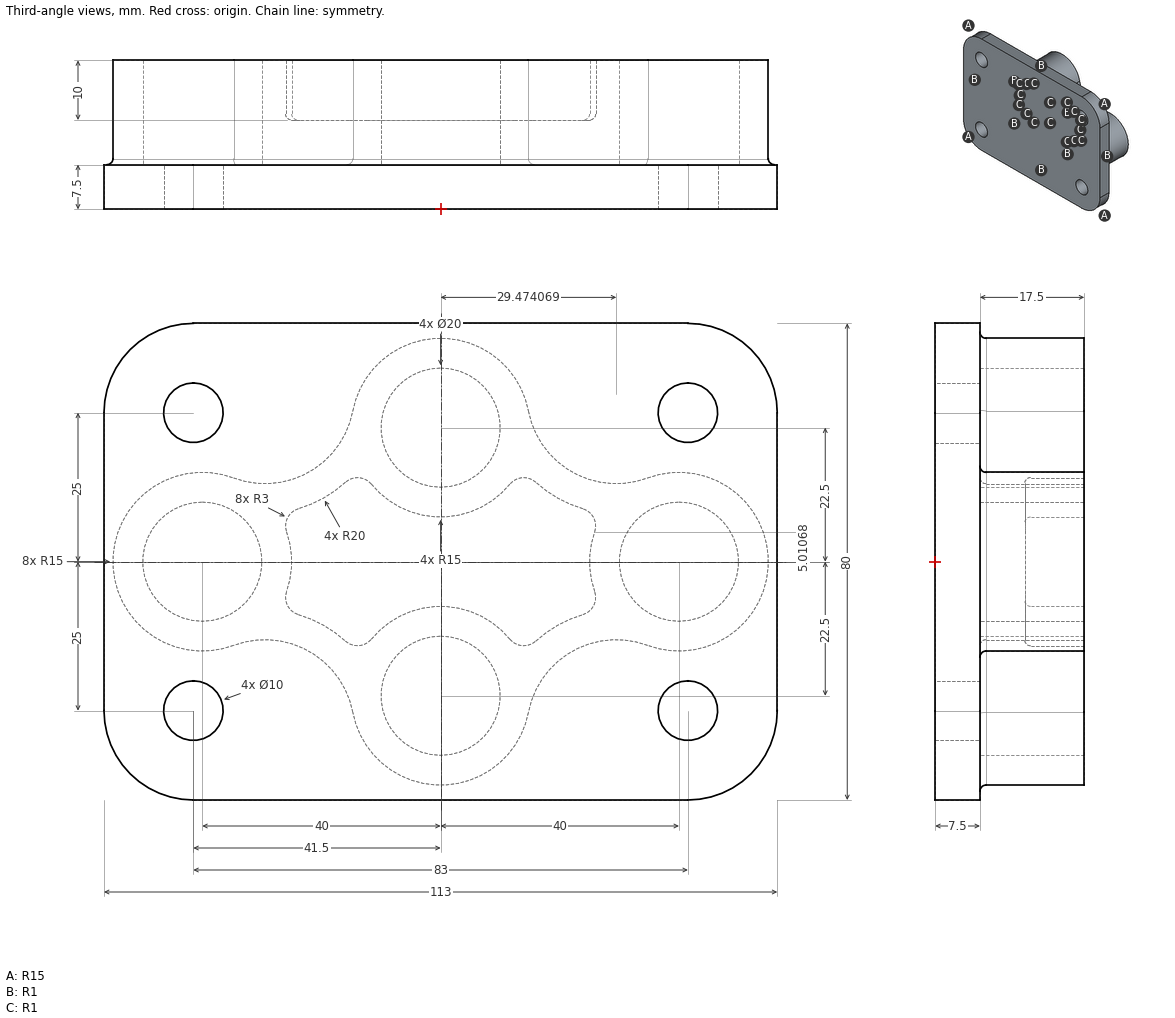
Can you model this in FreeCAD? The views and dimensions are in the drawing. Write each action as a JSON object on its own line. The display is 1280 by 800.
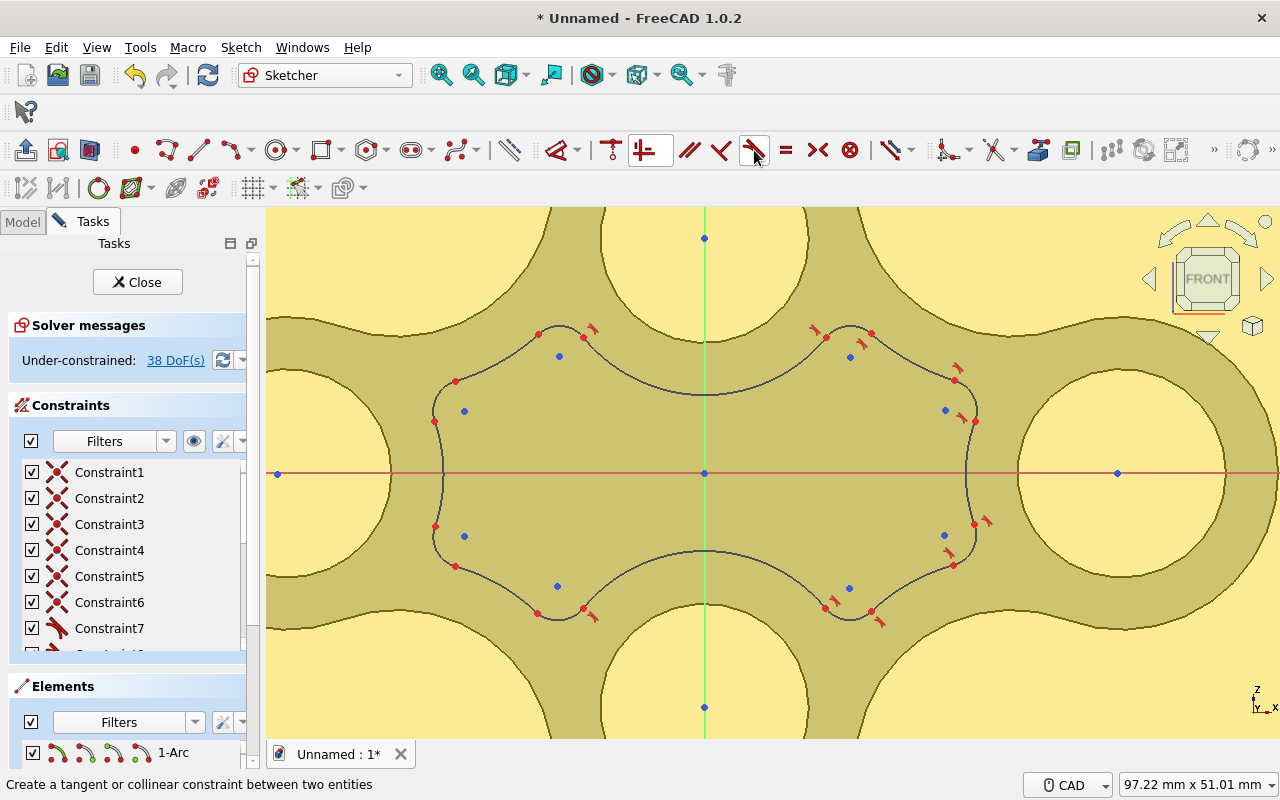
{"action": "left_click", "coordinate": [552, 620]}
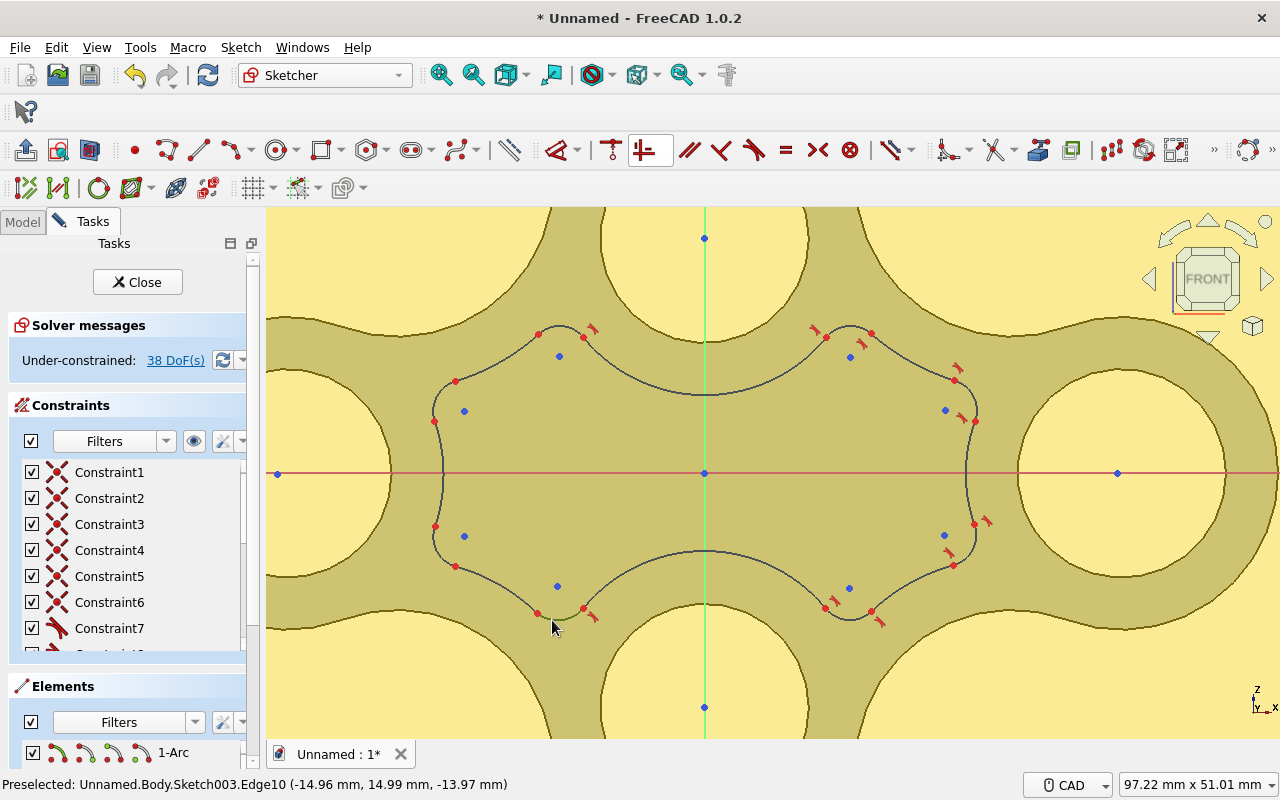
{"action": "left_click", "coordinate": [516, 595]}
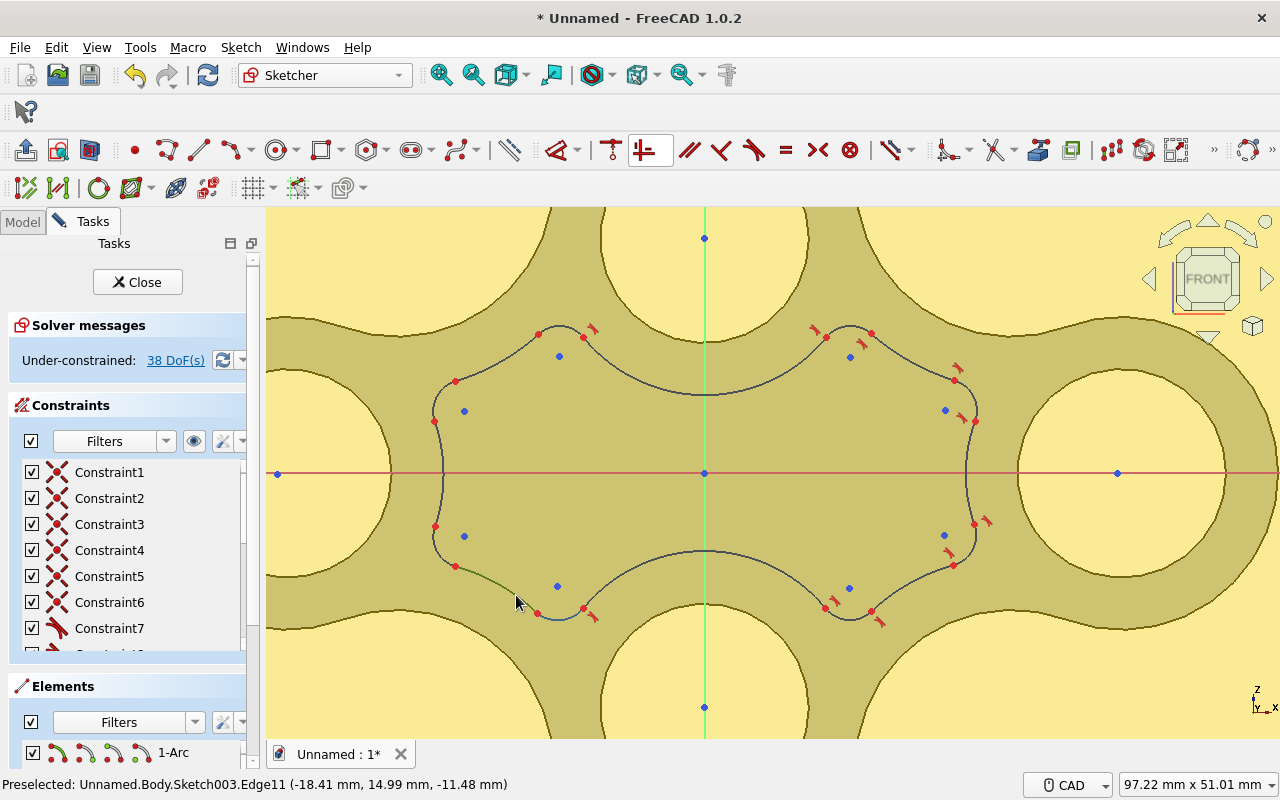
{"action": "key", "text": "t"}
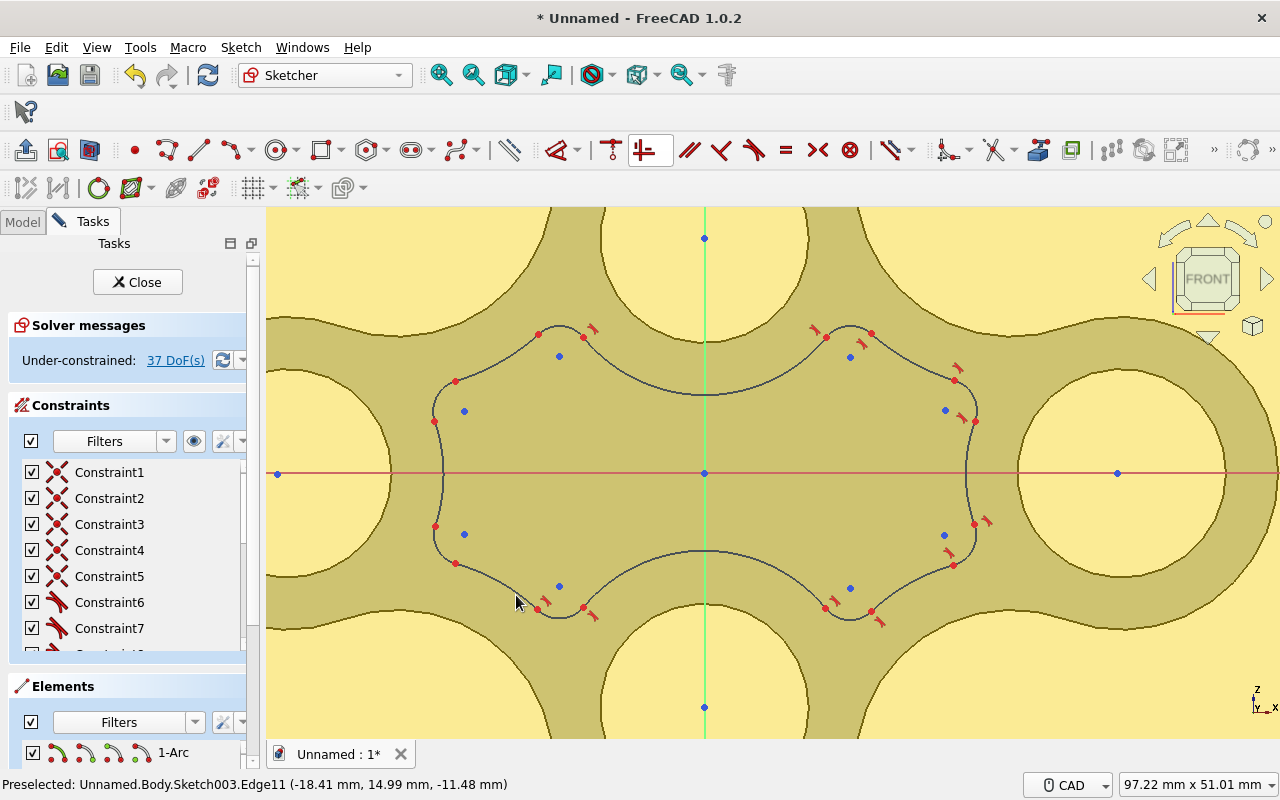
{"action": "left_click", "coordinate": [515, 592]}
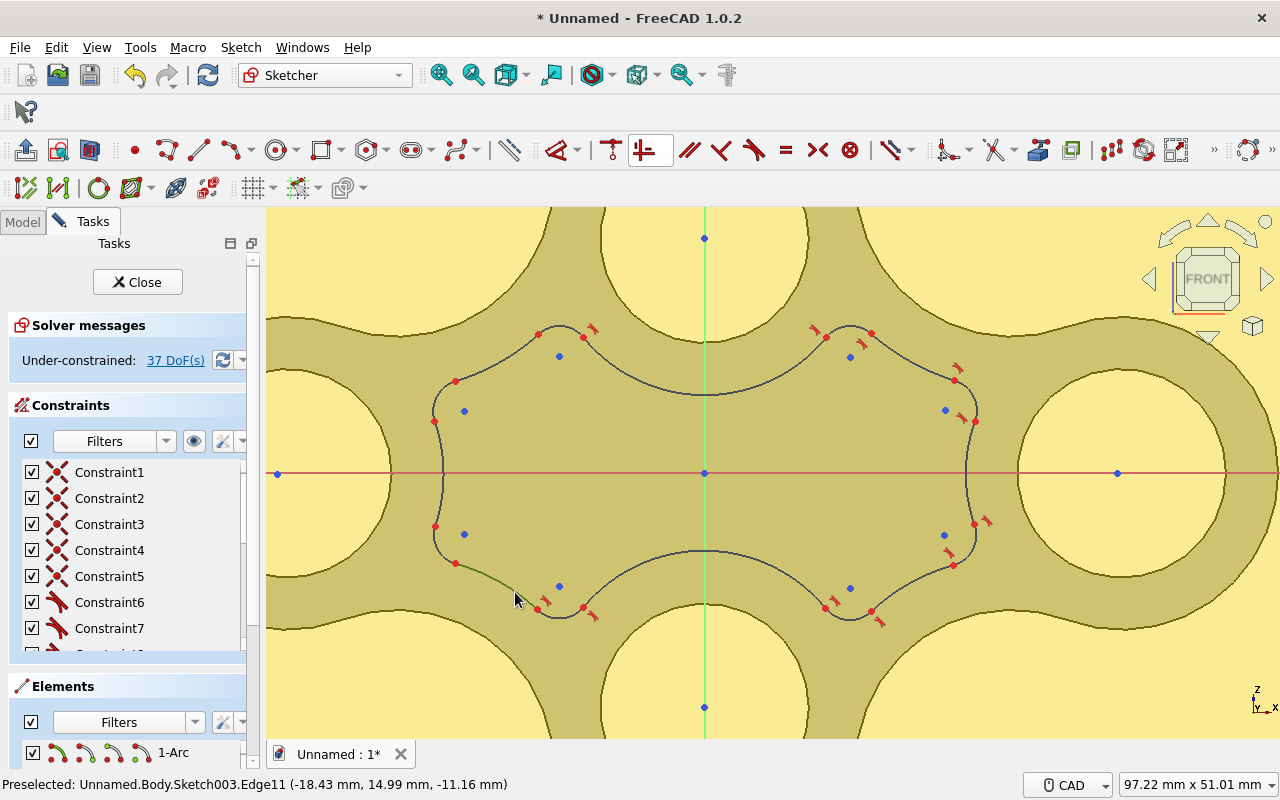
{"action": "left_click", "coordinate": [435, 541]}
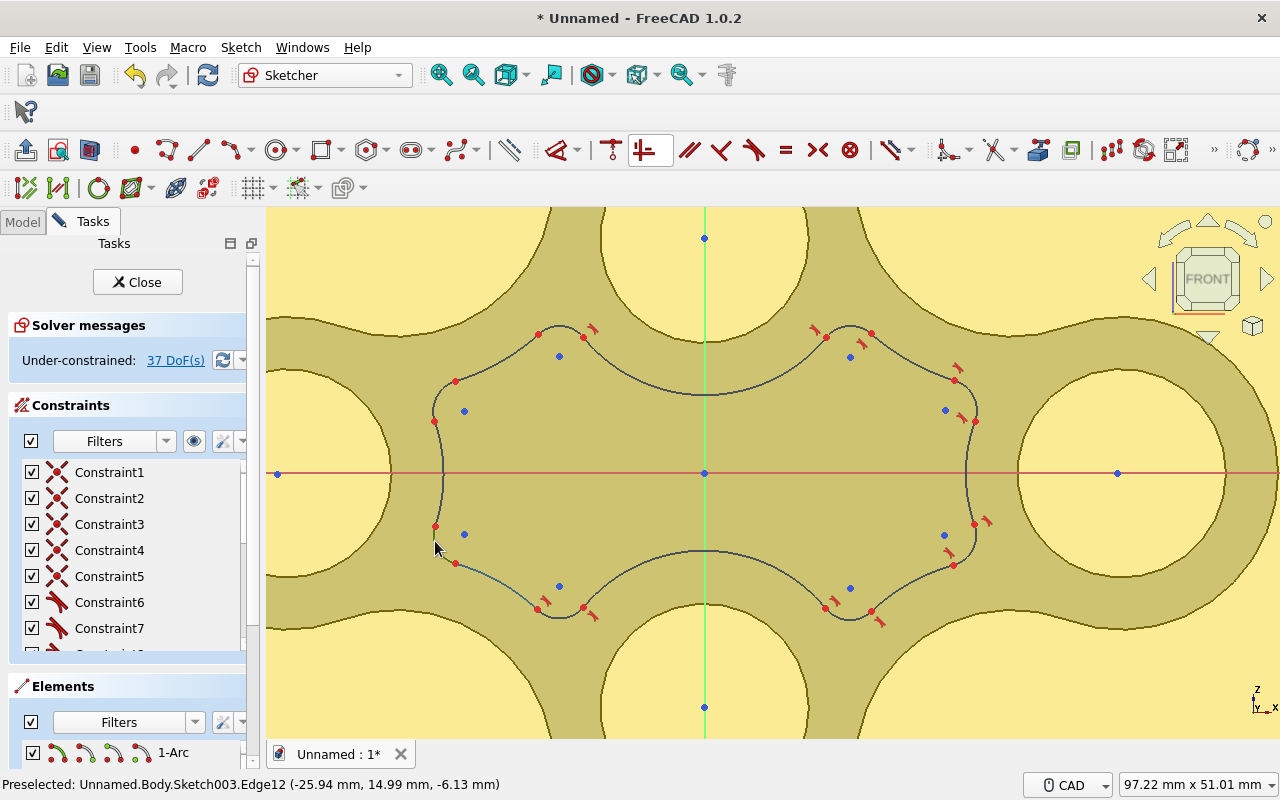
{"action": "key", "text": "t"}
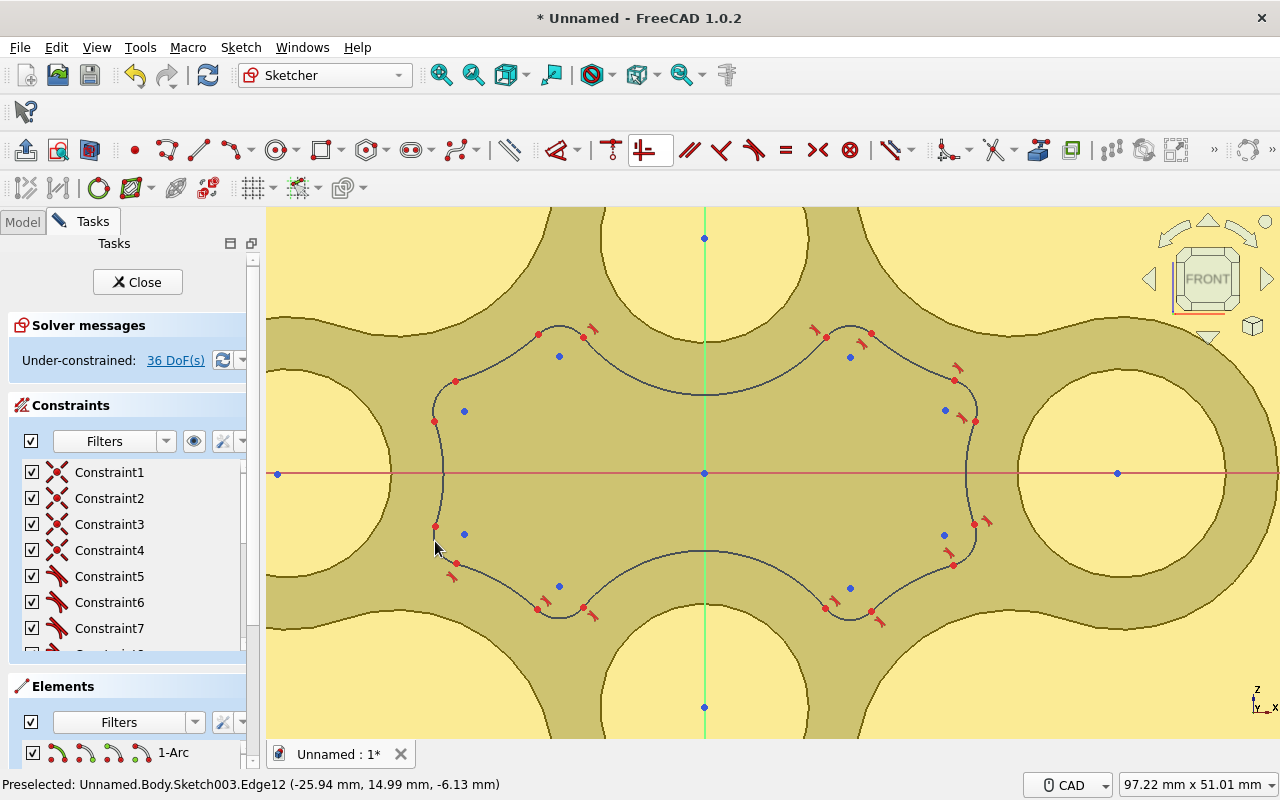
{"action": "left_click", "coordinate": [435, 541]}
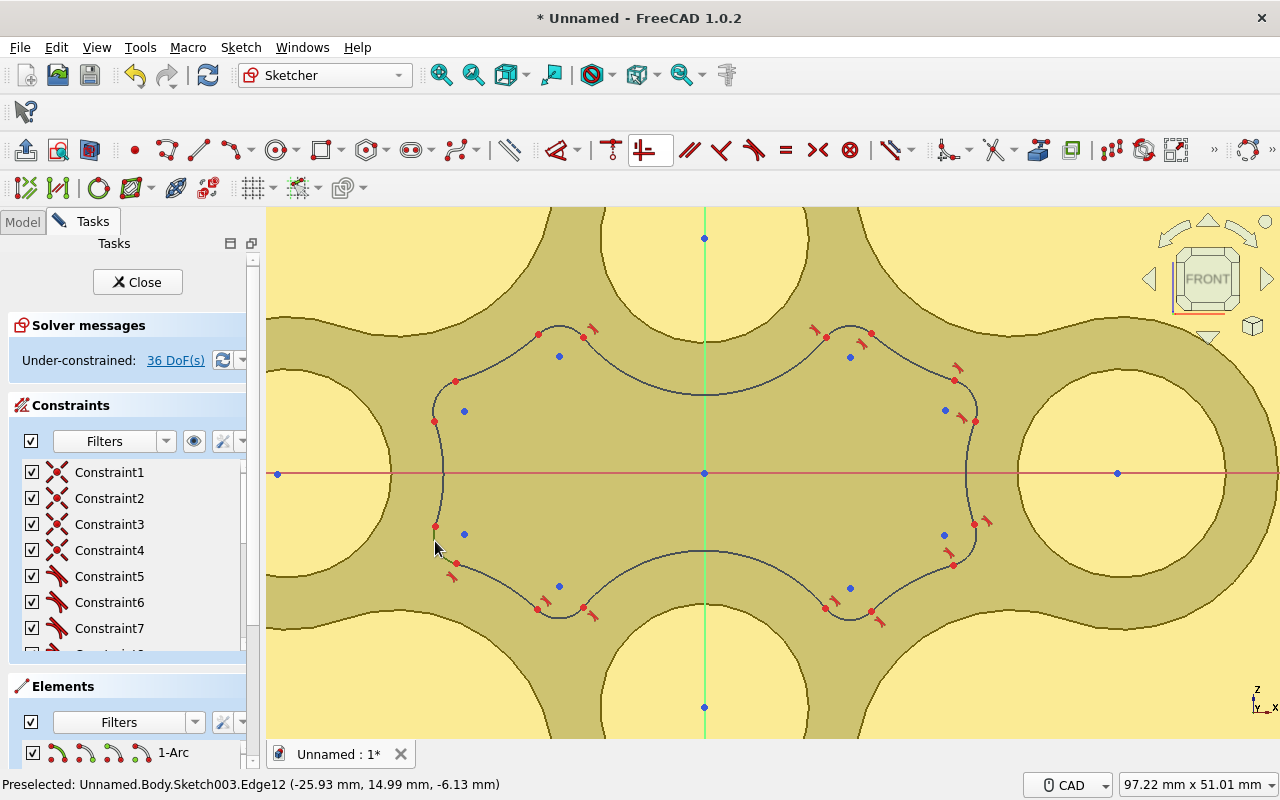
{"action": "left_click", "coordinate": [442, 496]}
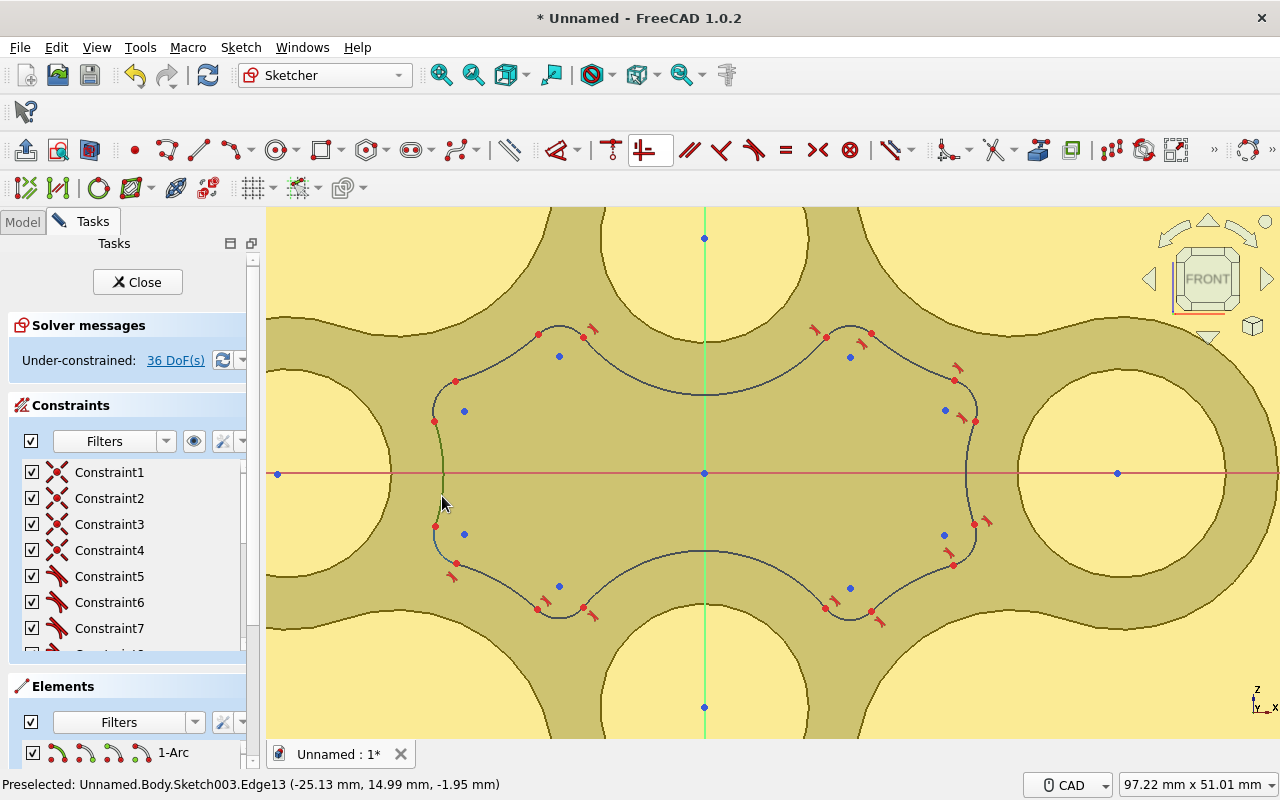
{"action": "key", "text": "t"}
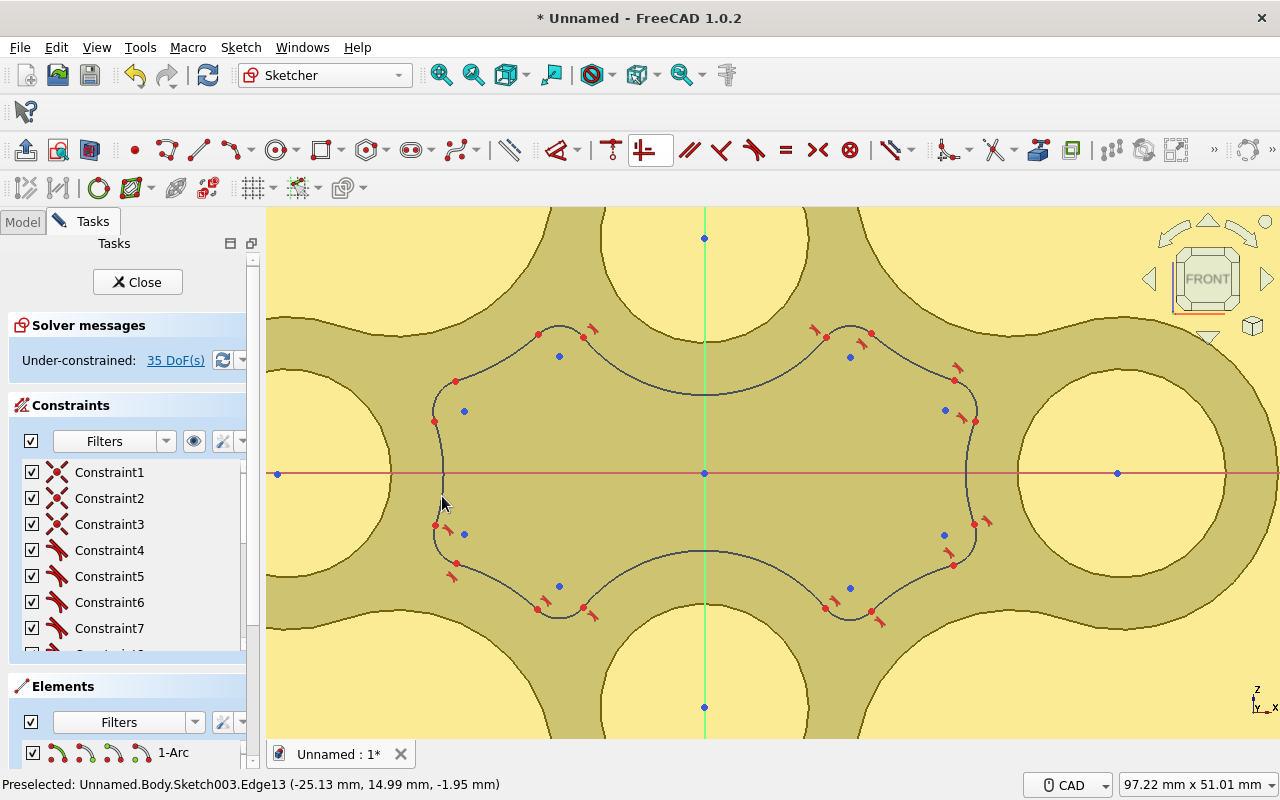
{"action": "left_click", "coordinate": [442, 495]}